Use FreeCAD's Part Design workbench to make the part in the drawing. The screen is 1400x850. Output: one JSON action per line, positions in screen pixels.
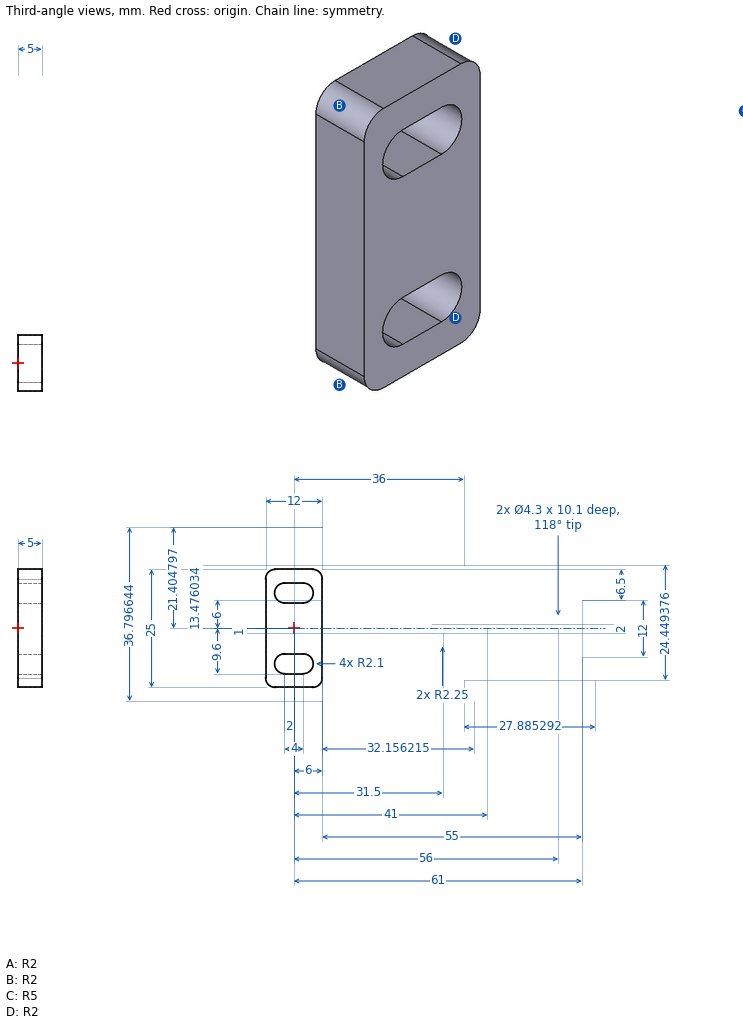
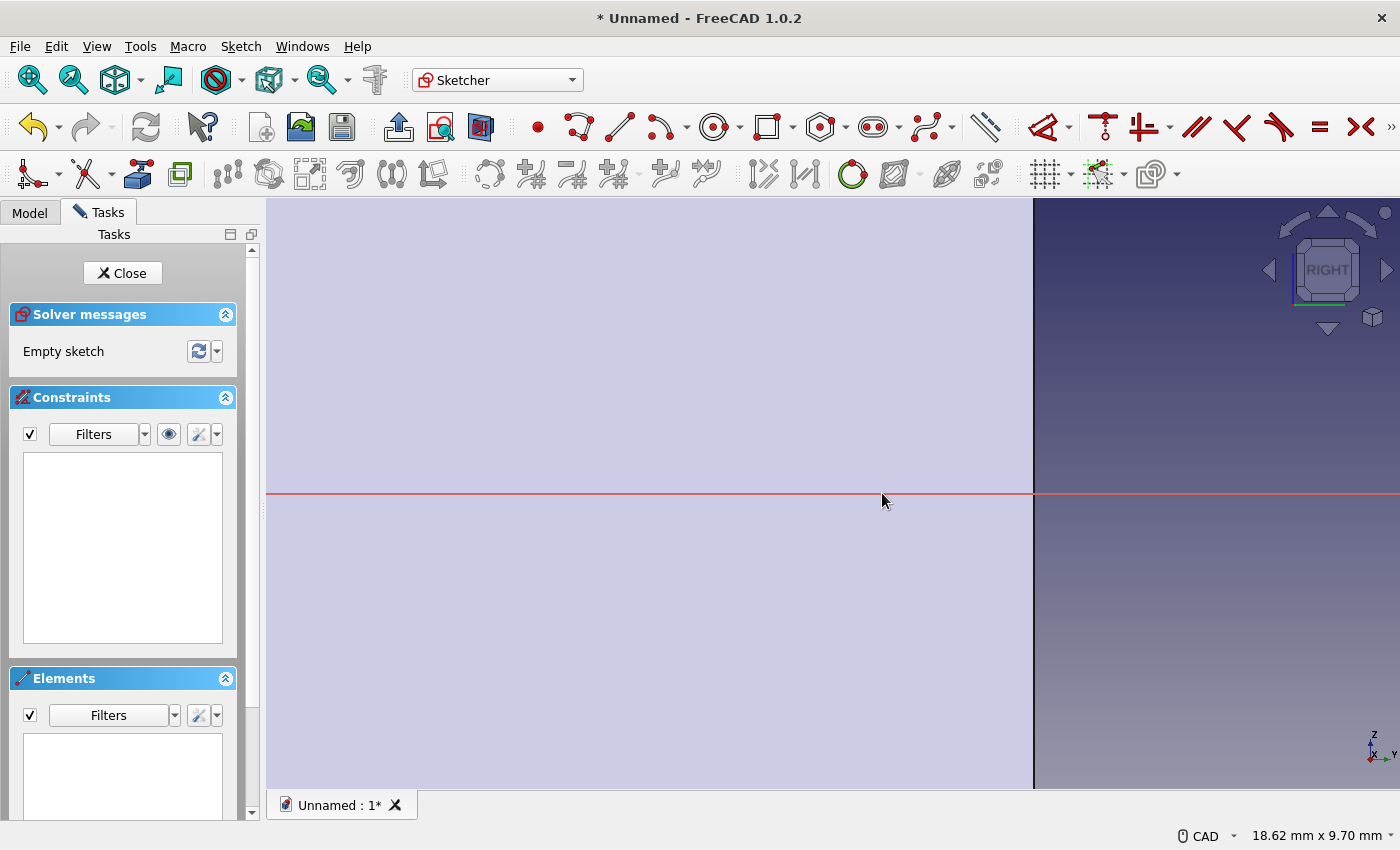
{"action": "left_click", "coordinate": [760, 554]}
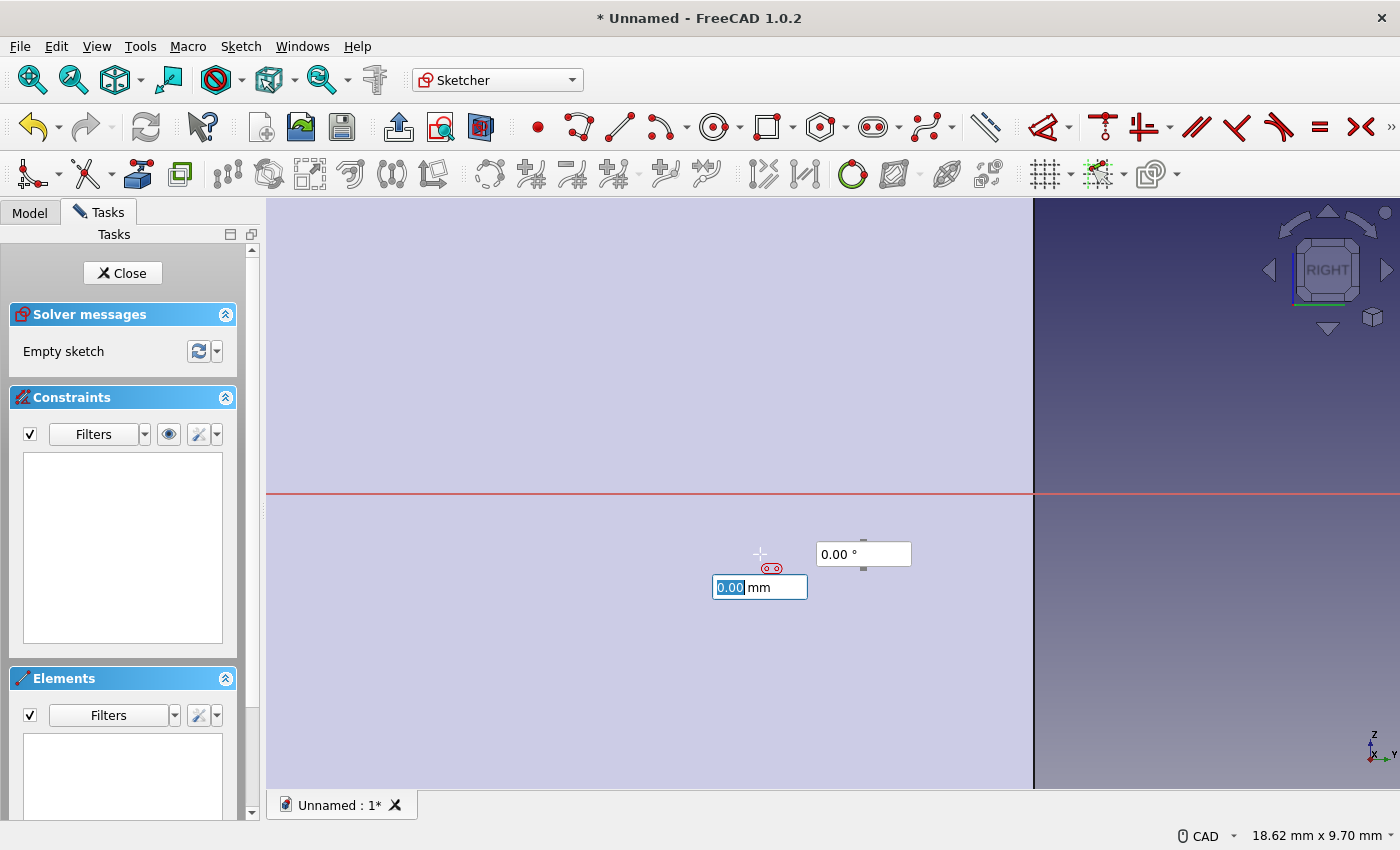
{"action": "left_click", "coordinate": [760, 433]}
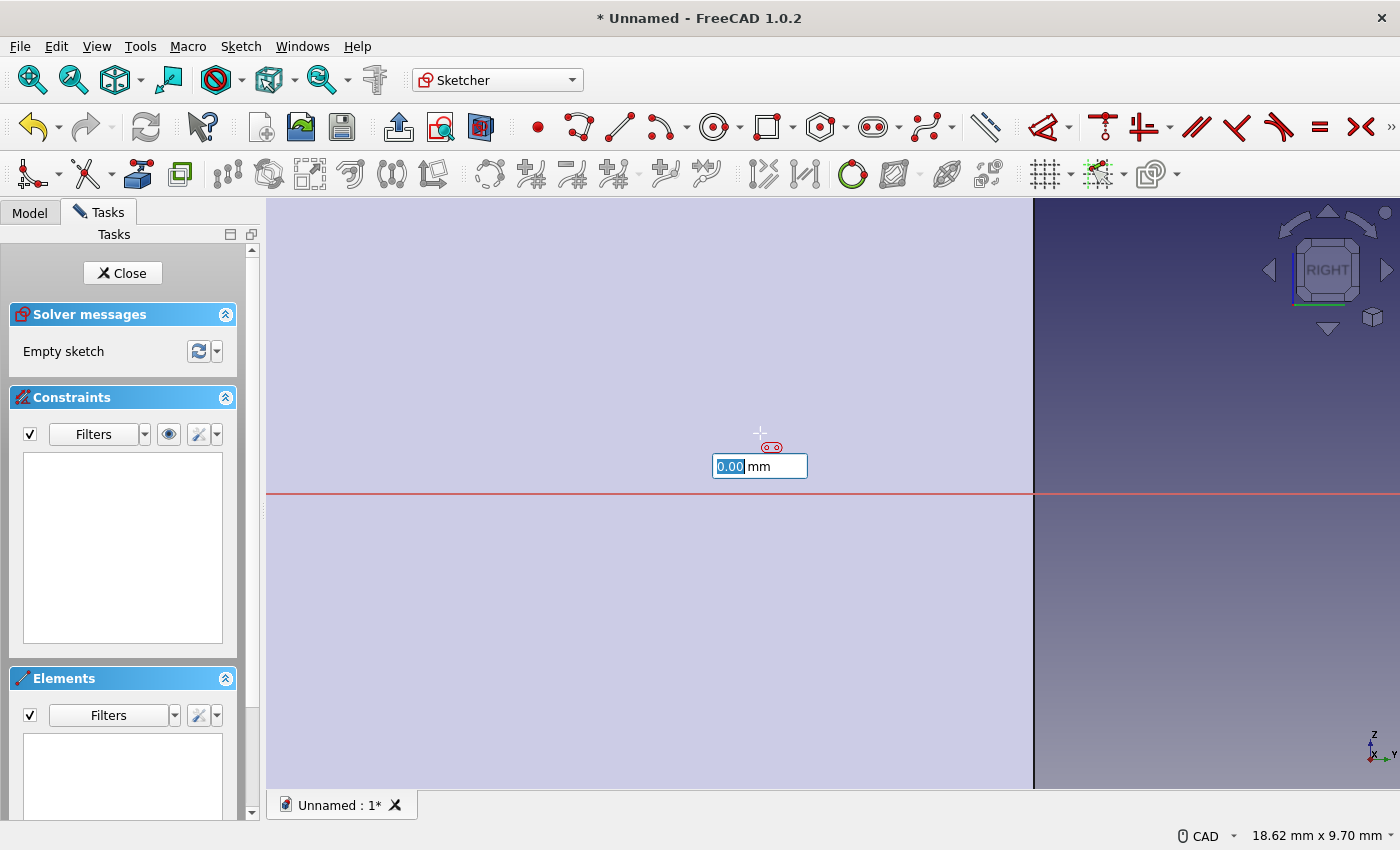
{"action": "left_click", "coordinate": [897, 475]}
{"action": "key", "text": "Escape"}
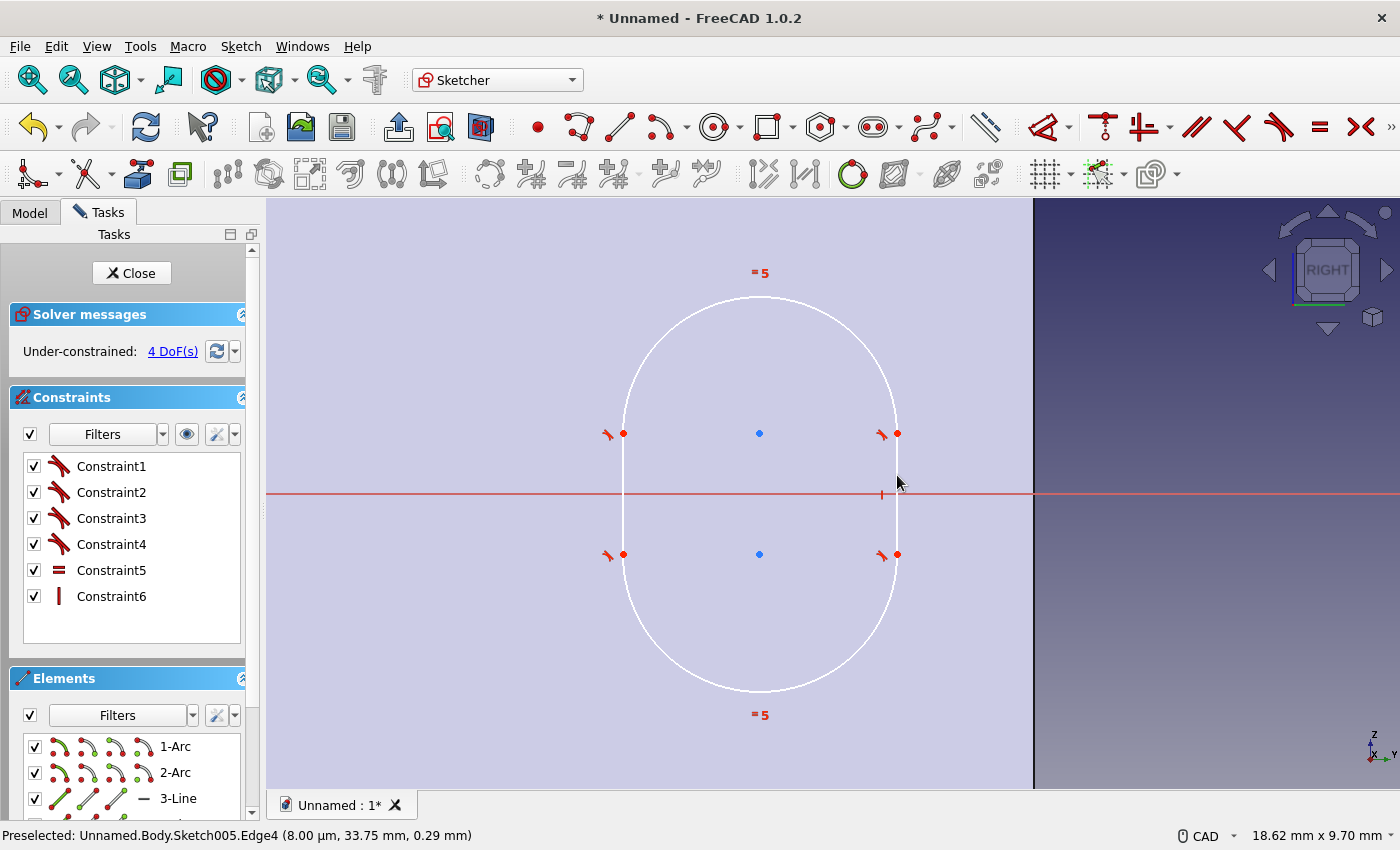
{"action": "left_click", "coordinate": [1042, 128]}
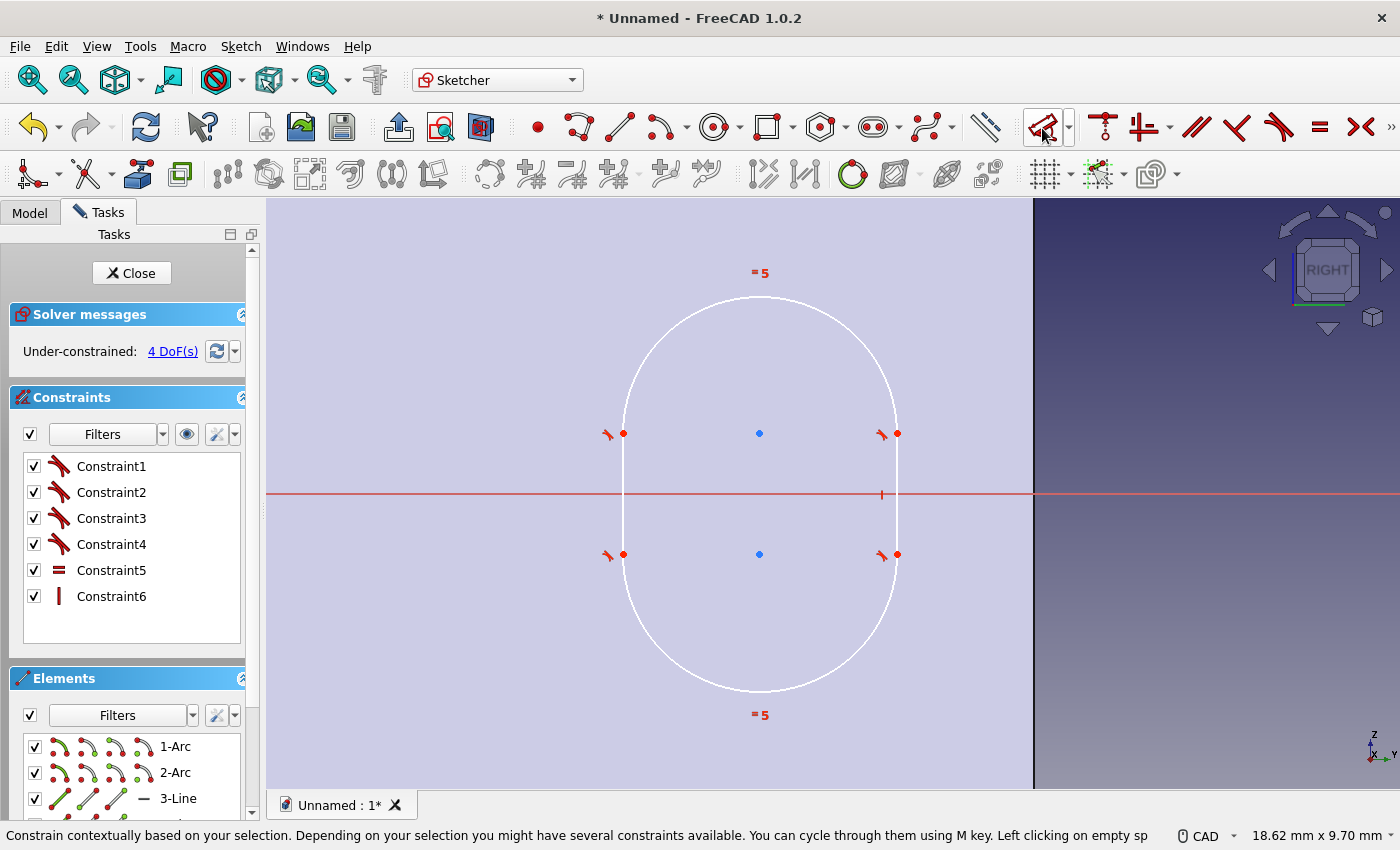
{"action": "left_click", "coordinate": [679, 666]}
{"action": "left_click", "coordinate": [660, 692]}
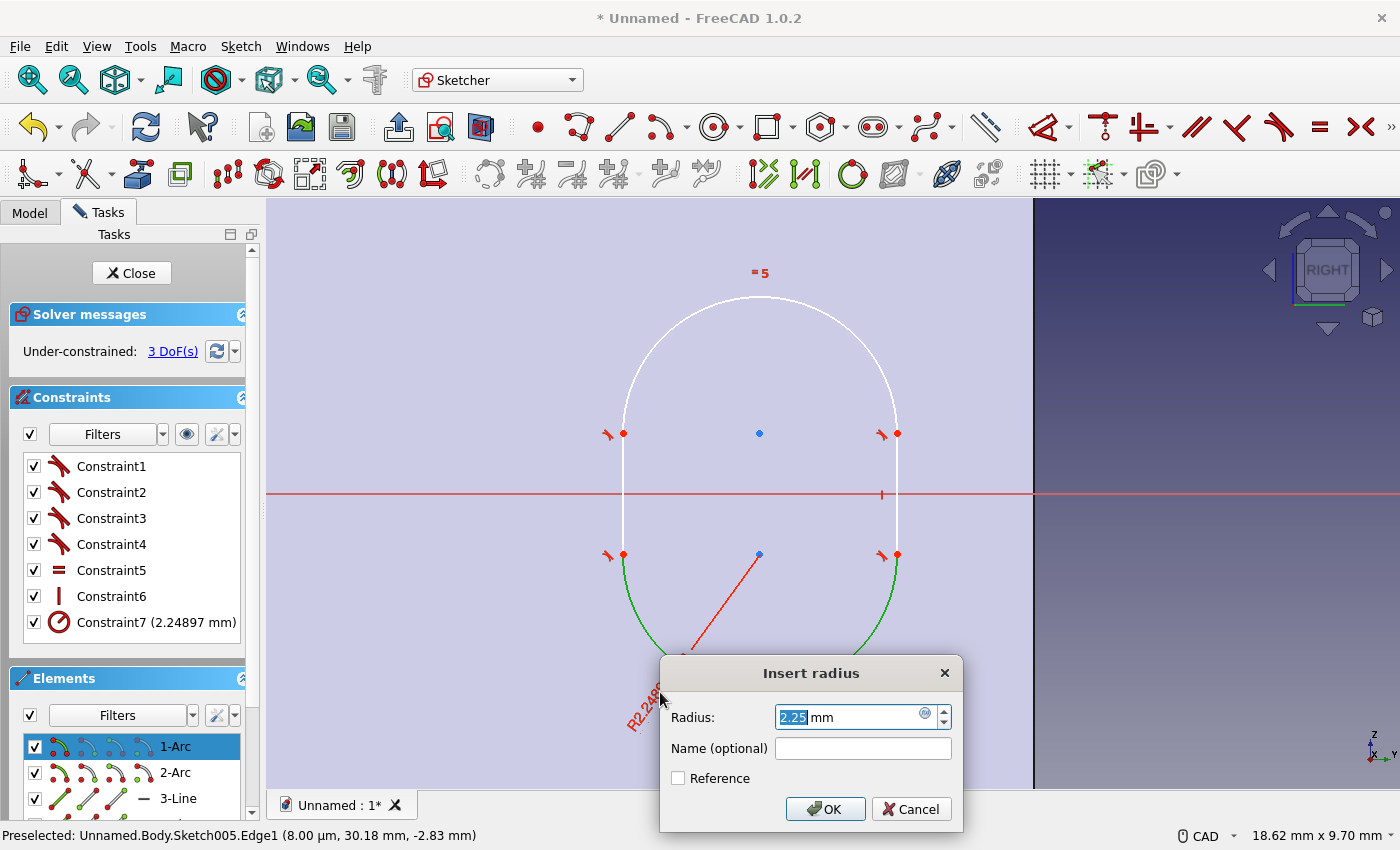
{"action": "type", "text": "2.25"}
{"action": "key", "text": "Return"}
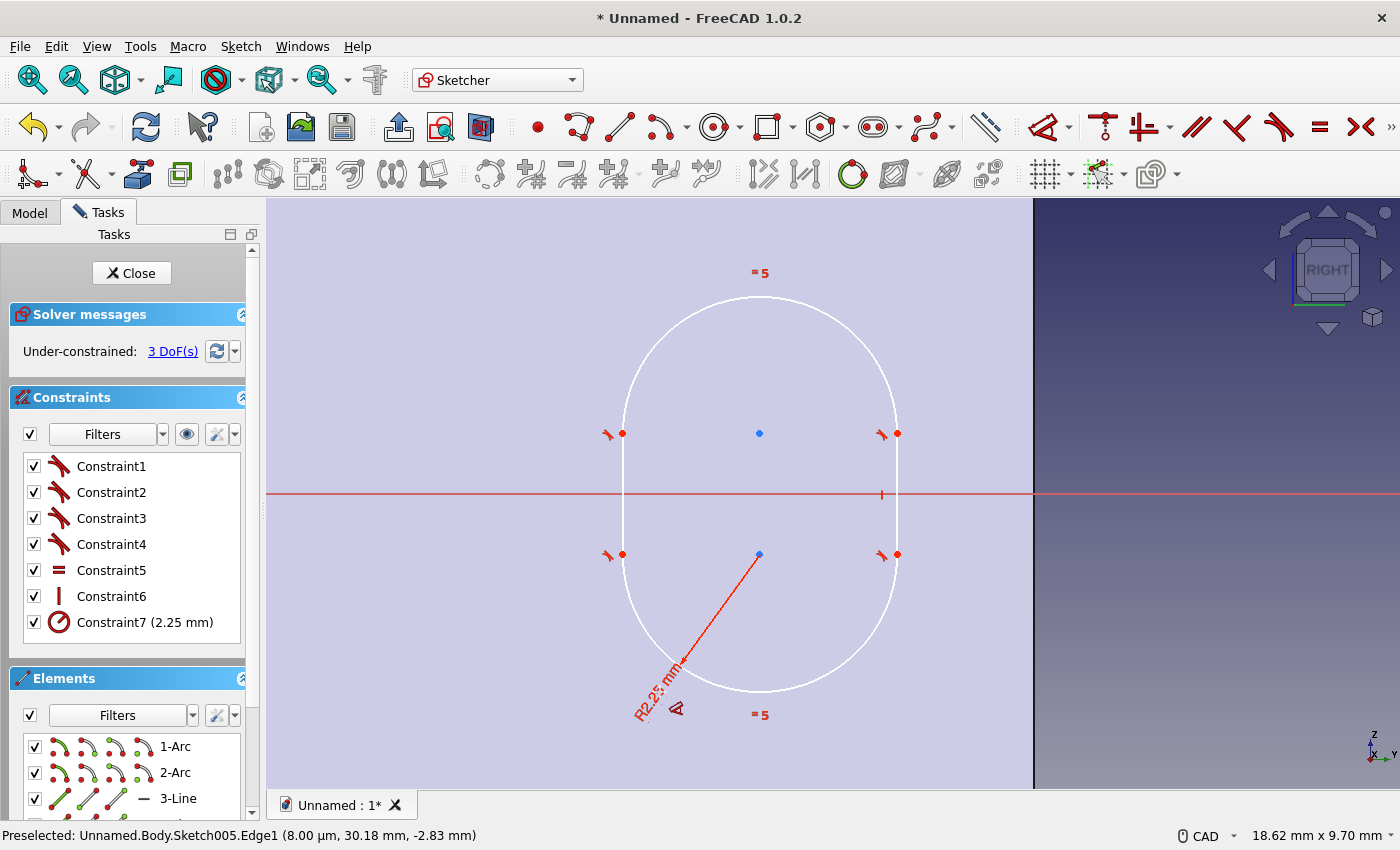
{"action": "left_click", "coordinate": [623, 519]}
{"action": "left_click", "coordinate": [589, 467]}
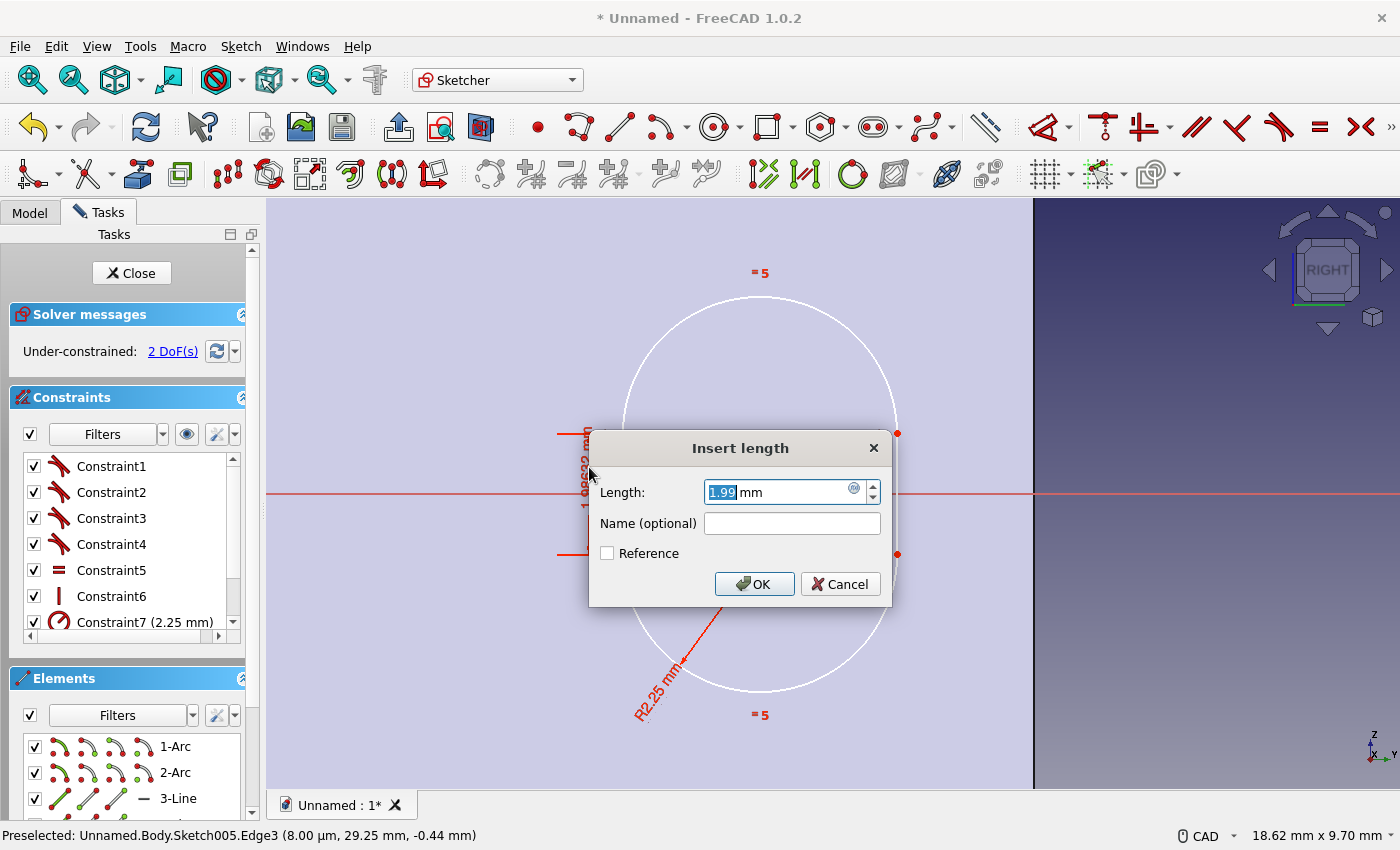
{"action": "type", "text": "2"}
{"action": "key", "text": "Return"}